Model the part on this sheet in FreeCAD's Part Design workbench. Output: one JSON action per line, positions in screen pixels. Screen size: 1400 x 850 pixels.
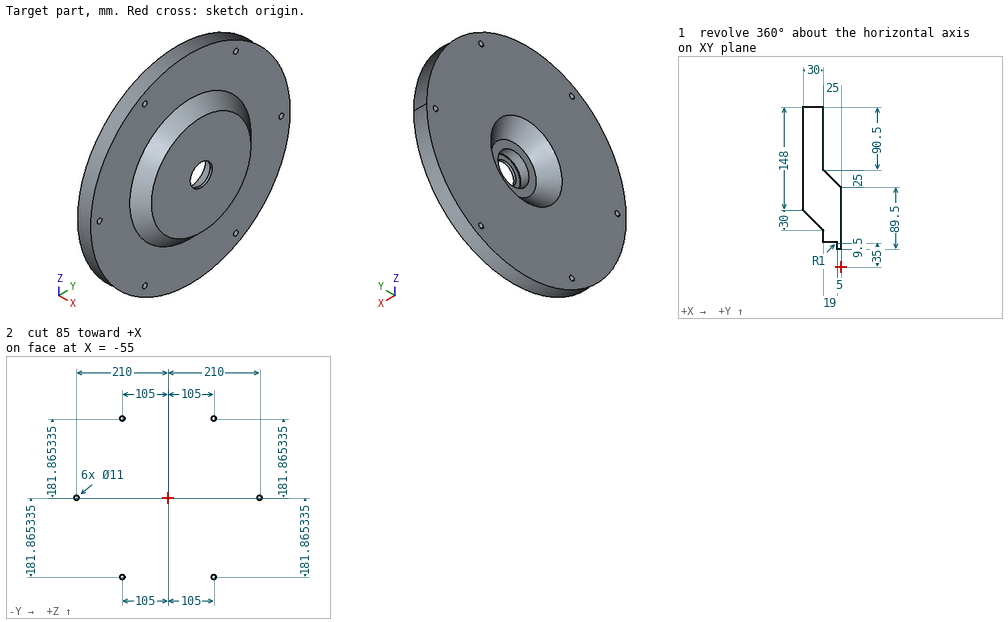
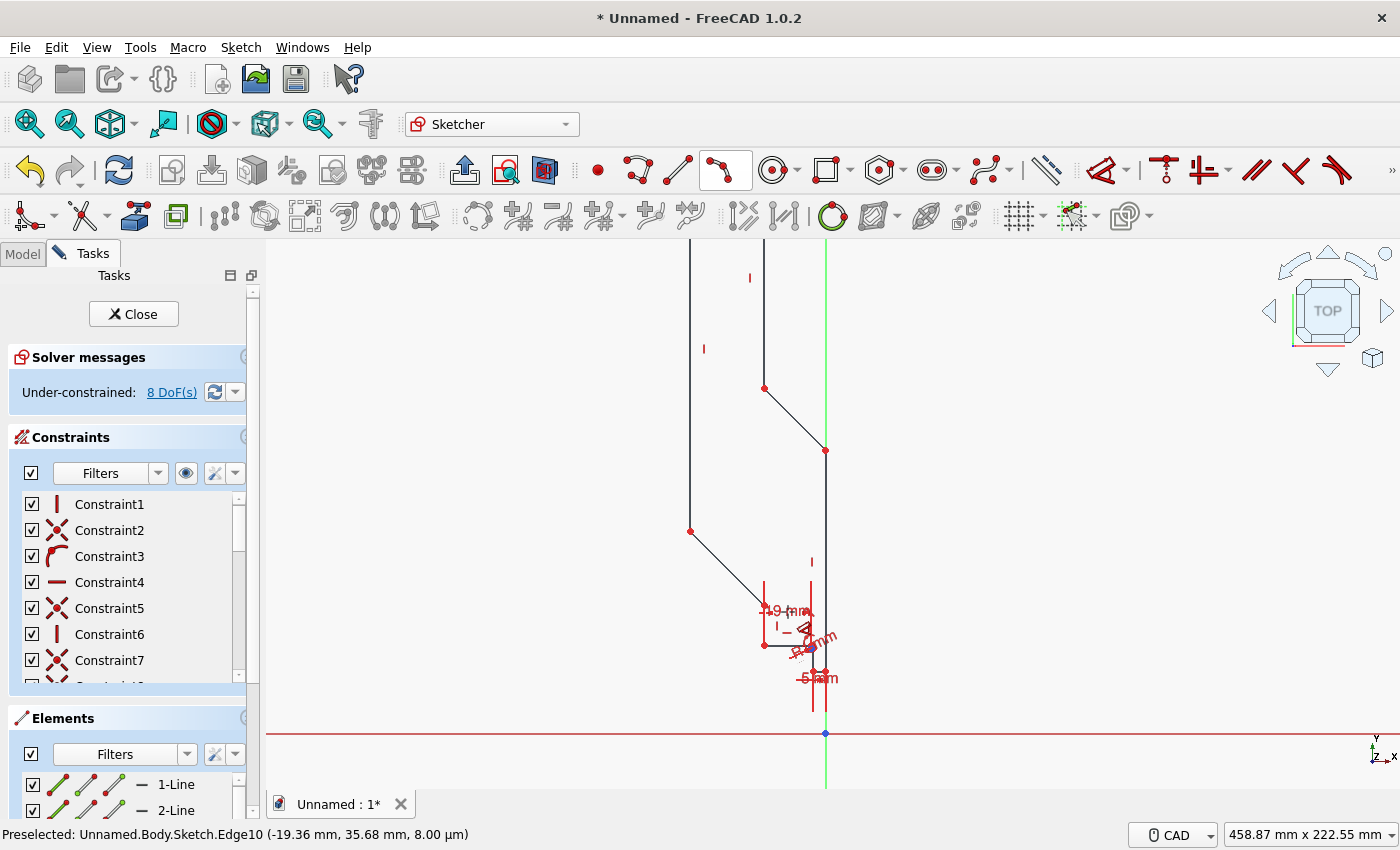
{"action": "scroll", "coordinate": [813, 658], "scroll_direction": "up", "scroll_amount": 3}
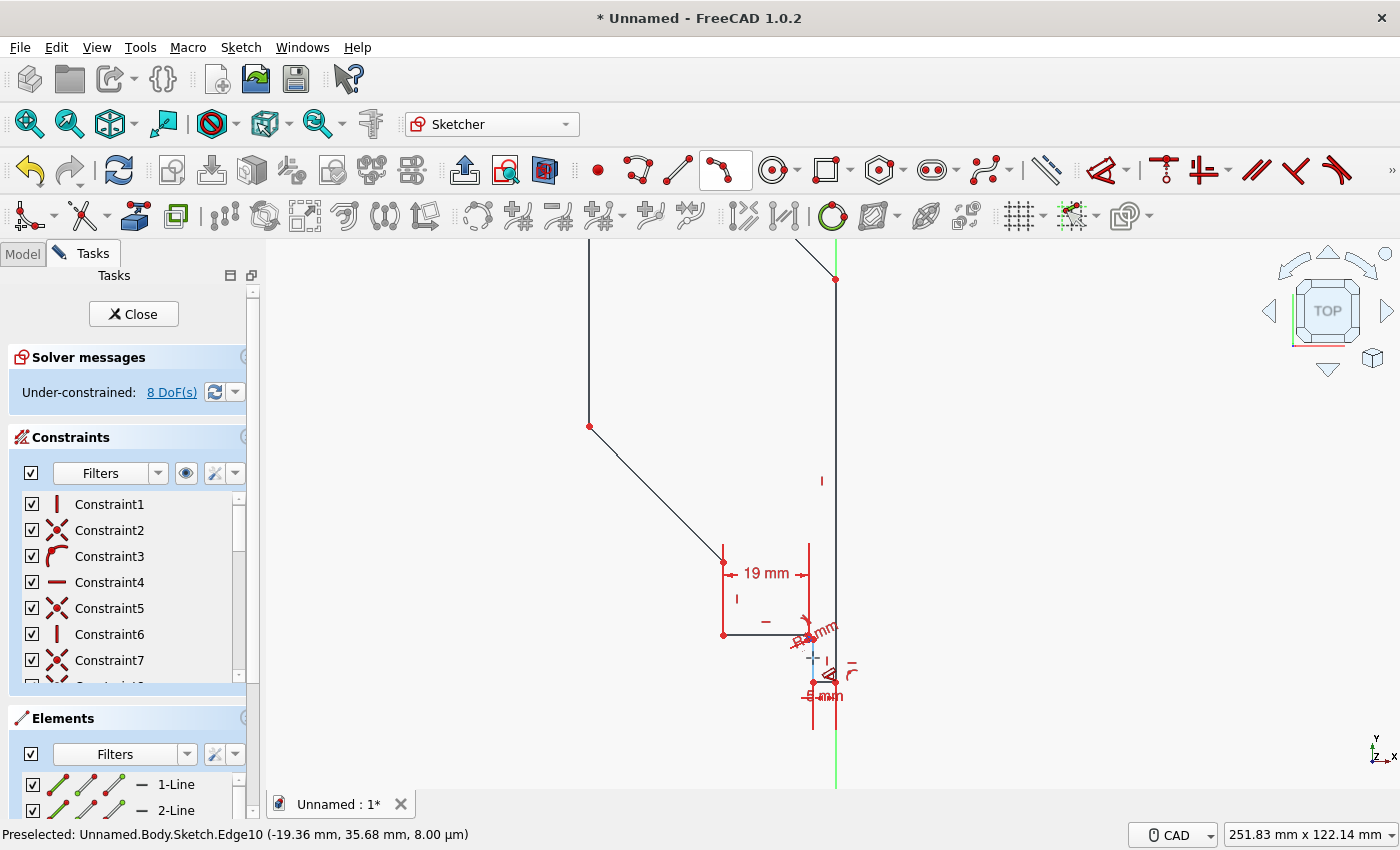
{"action": "left_click", "coordinate": [813, 657]}
{"action": "left_click", "coordinate": [779, 661]}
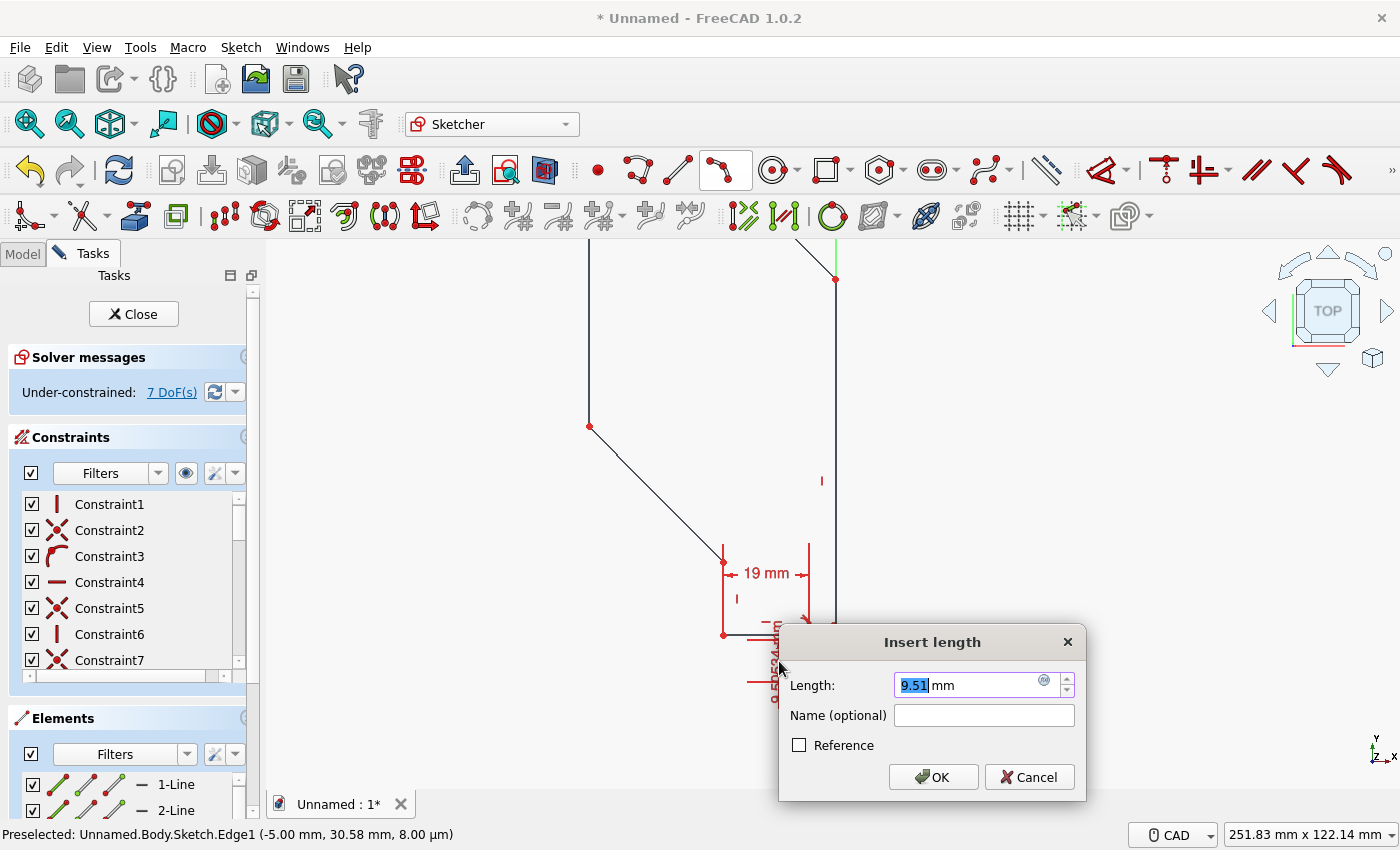
{"action": "type", "text": "9.5"}
{"action": "key", "text": "Return"}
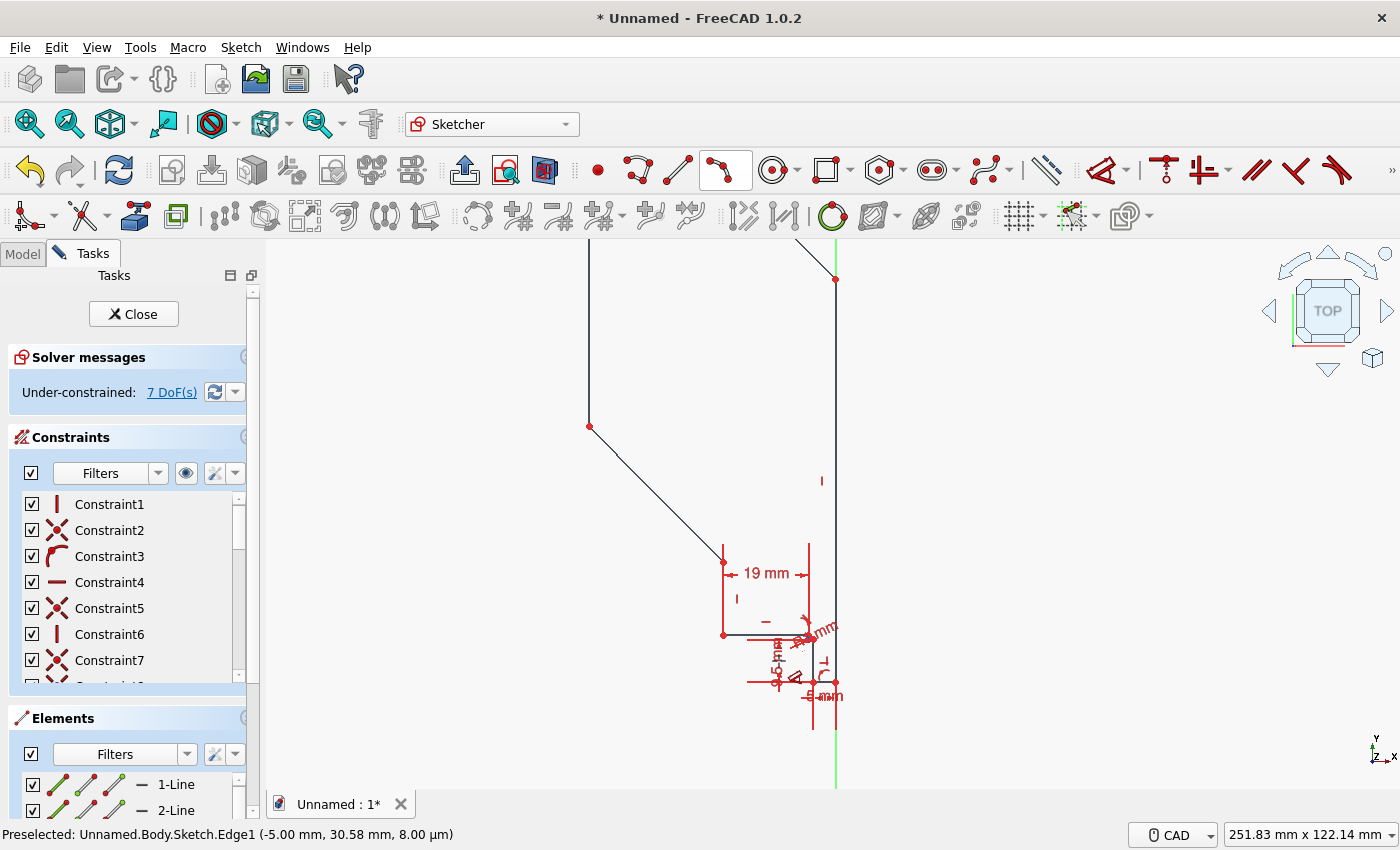
{"action": "left_click", "coordinate": [589, 294]}
{"action": "left_click", "coordinate": [555, 347]}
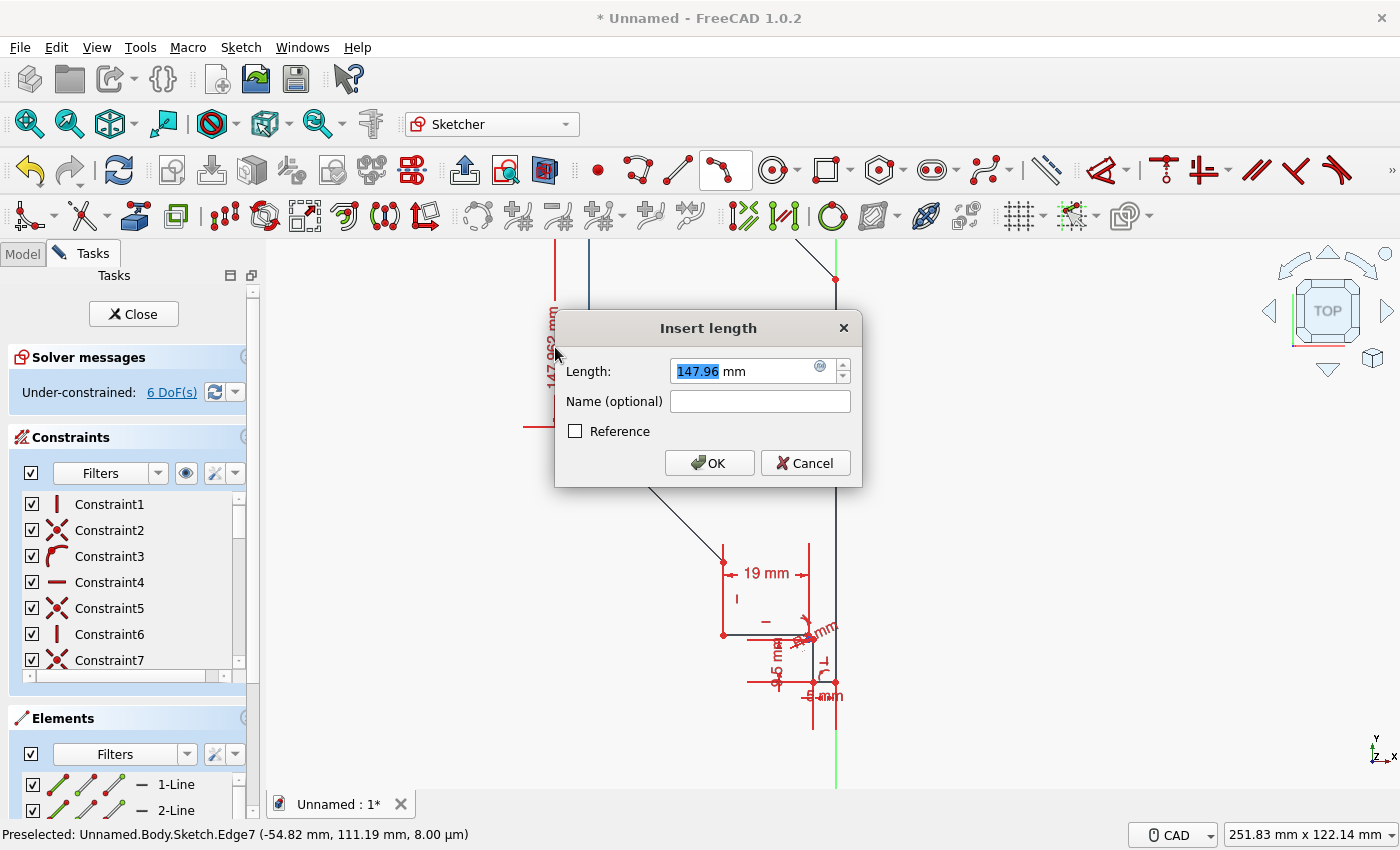
{"action": "type", "text": "148"}
{"action": "key", "text": "Return"}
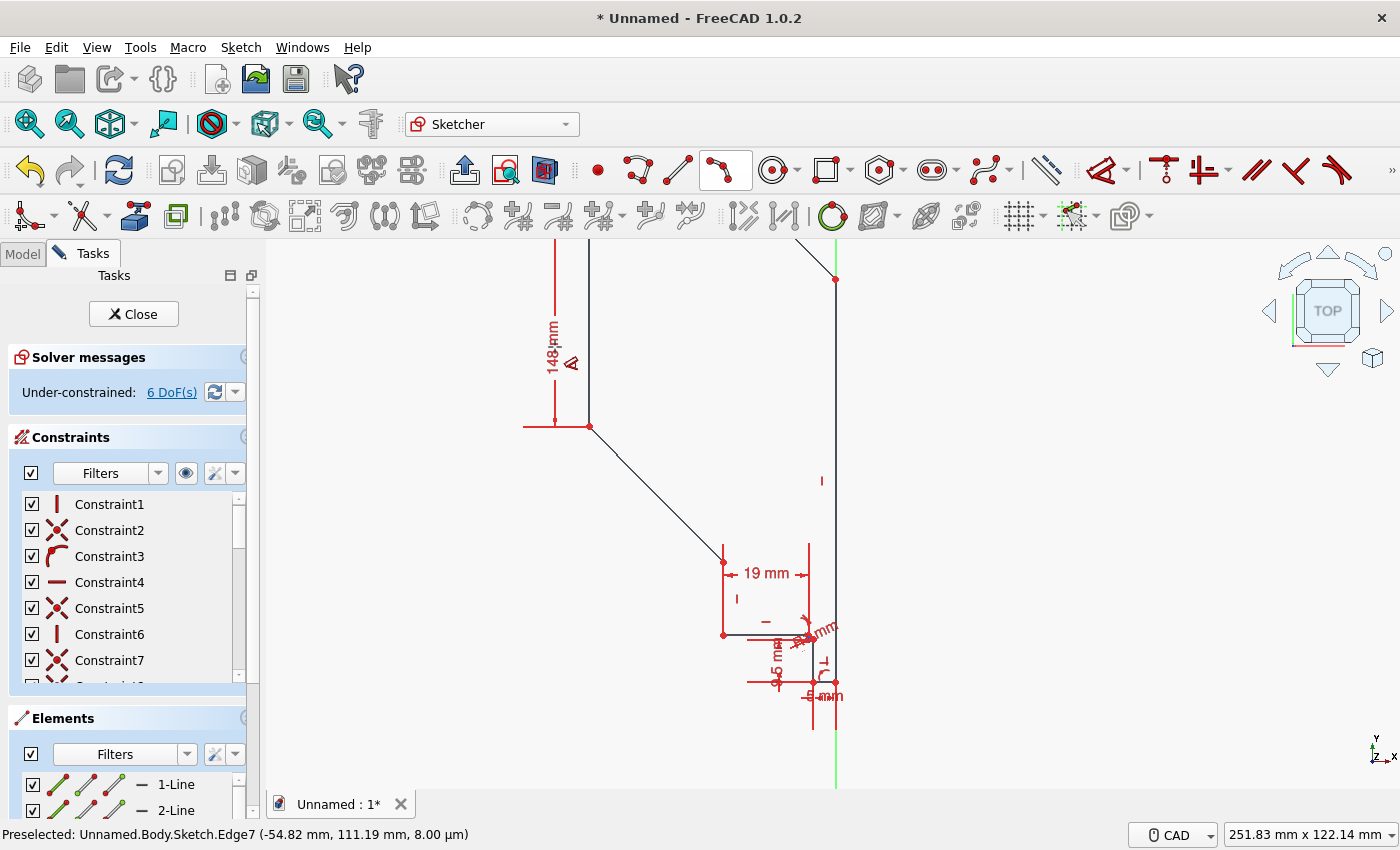
{"action": "scroll", "coordinate": [813, 640], "scroll_direction": "up", "scroll_amount": 5}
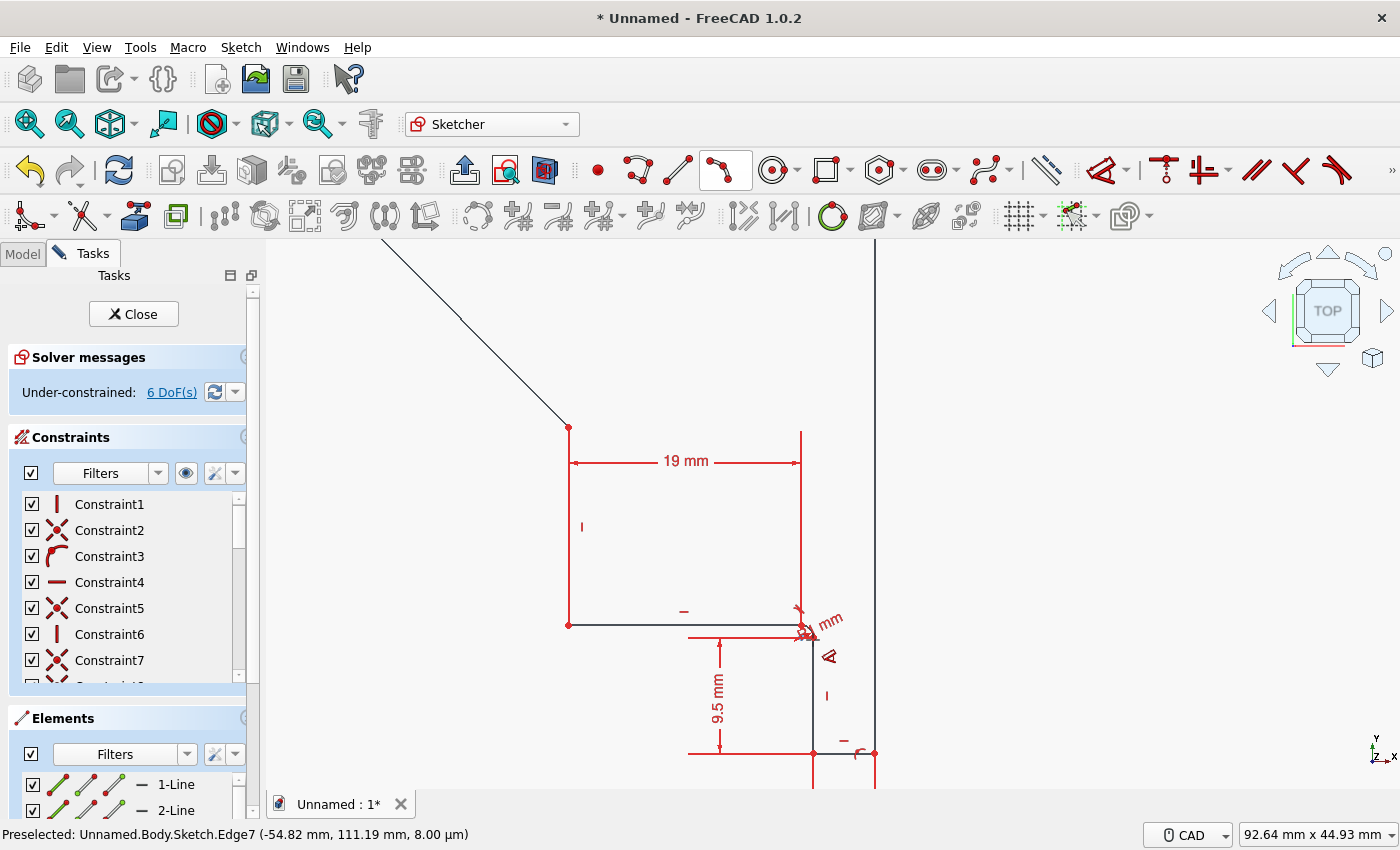
{"action": "left_click", "coordinate": [813, 638]}
{"action": "left_click", "coordinate": [909, 699]}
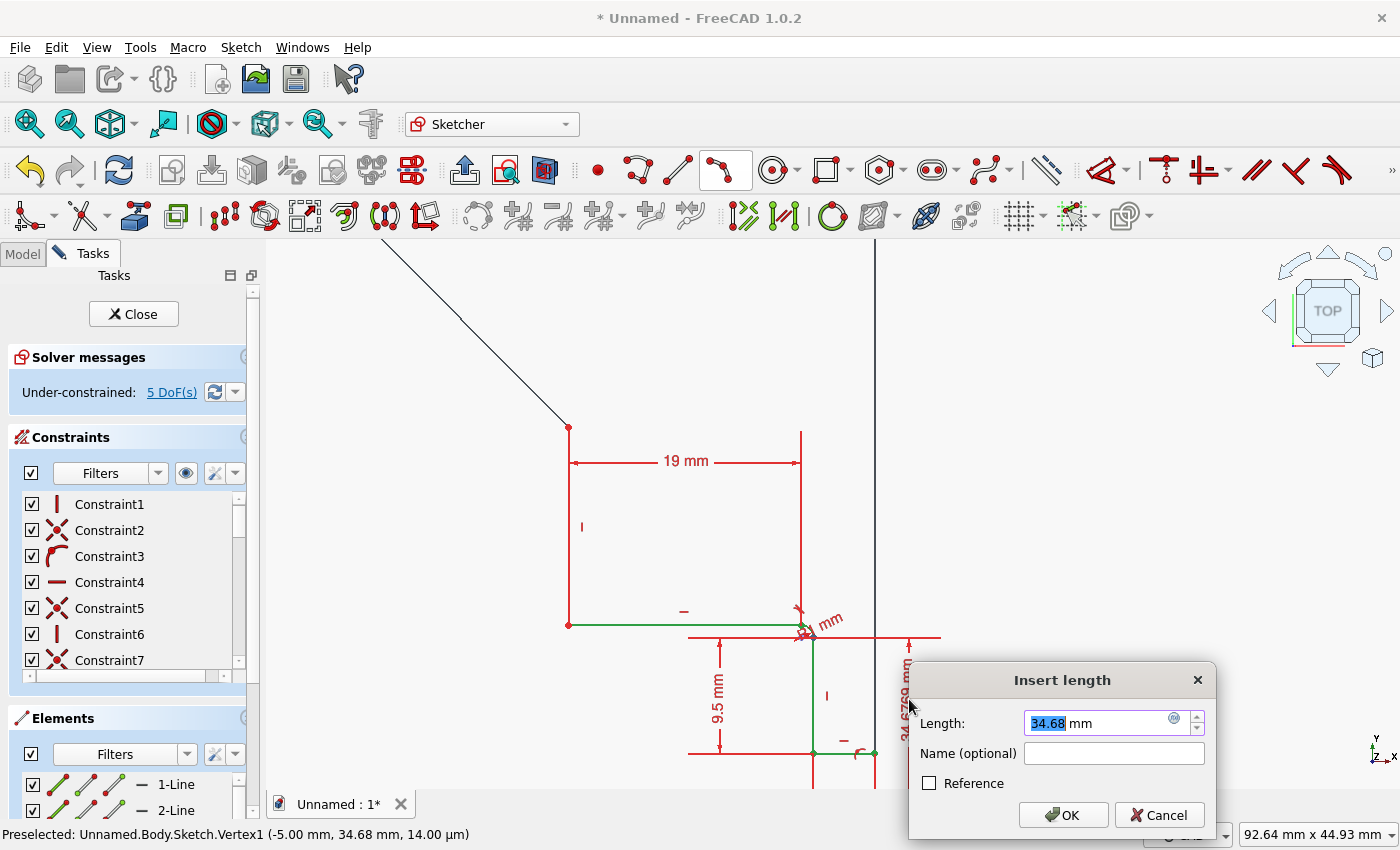
{"action": "type", "text": "35"}
{"action": "key", "text": "Return"}